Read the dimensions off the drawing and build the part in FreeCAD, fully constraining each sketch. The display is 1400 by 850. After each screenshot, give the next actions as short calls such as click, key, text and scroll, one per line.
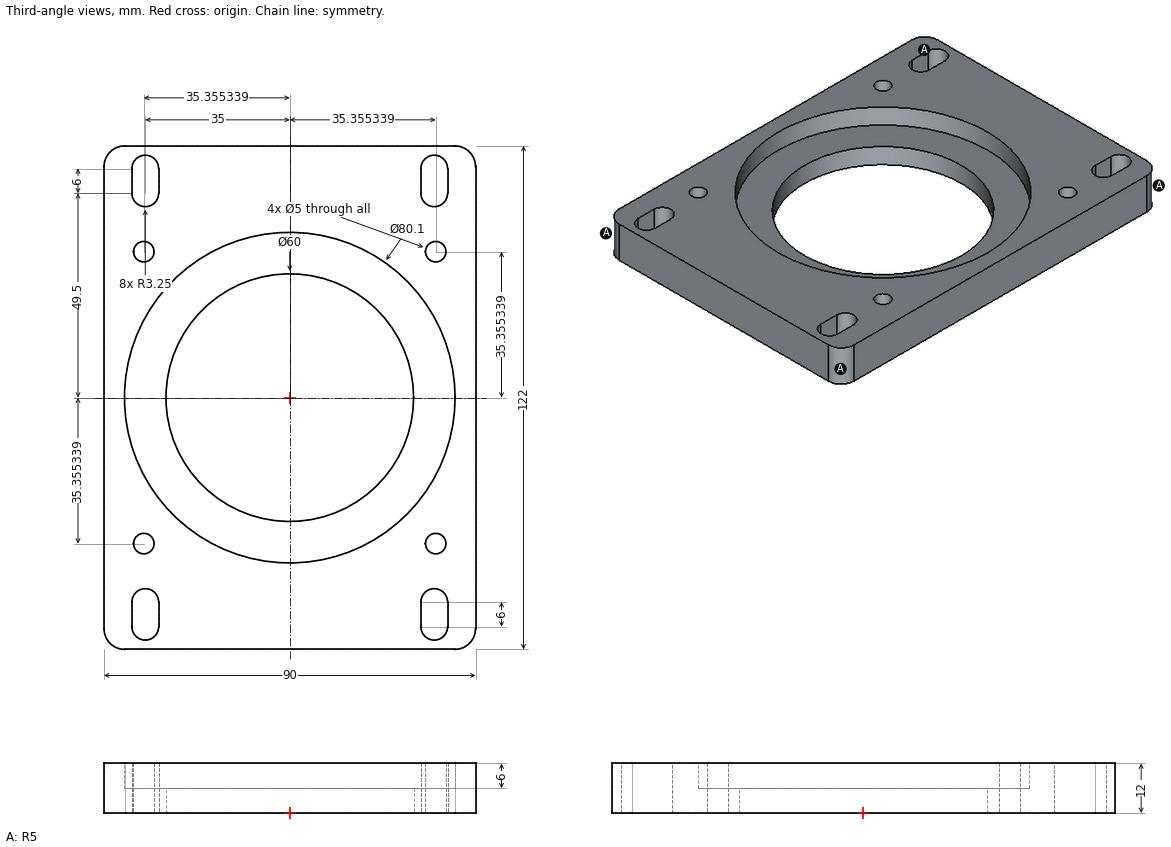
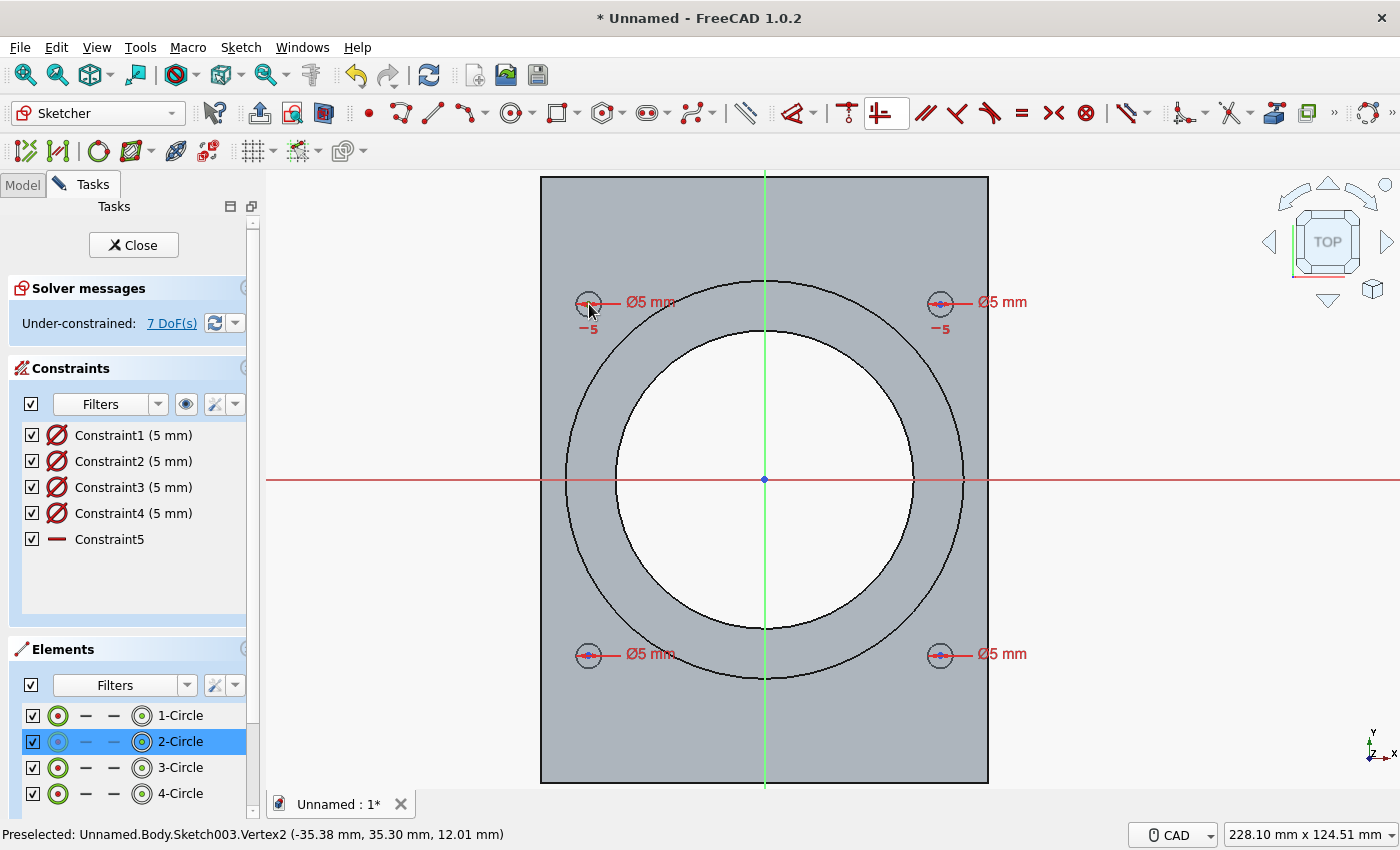
click(589, 656)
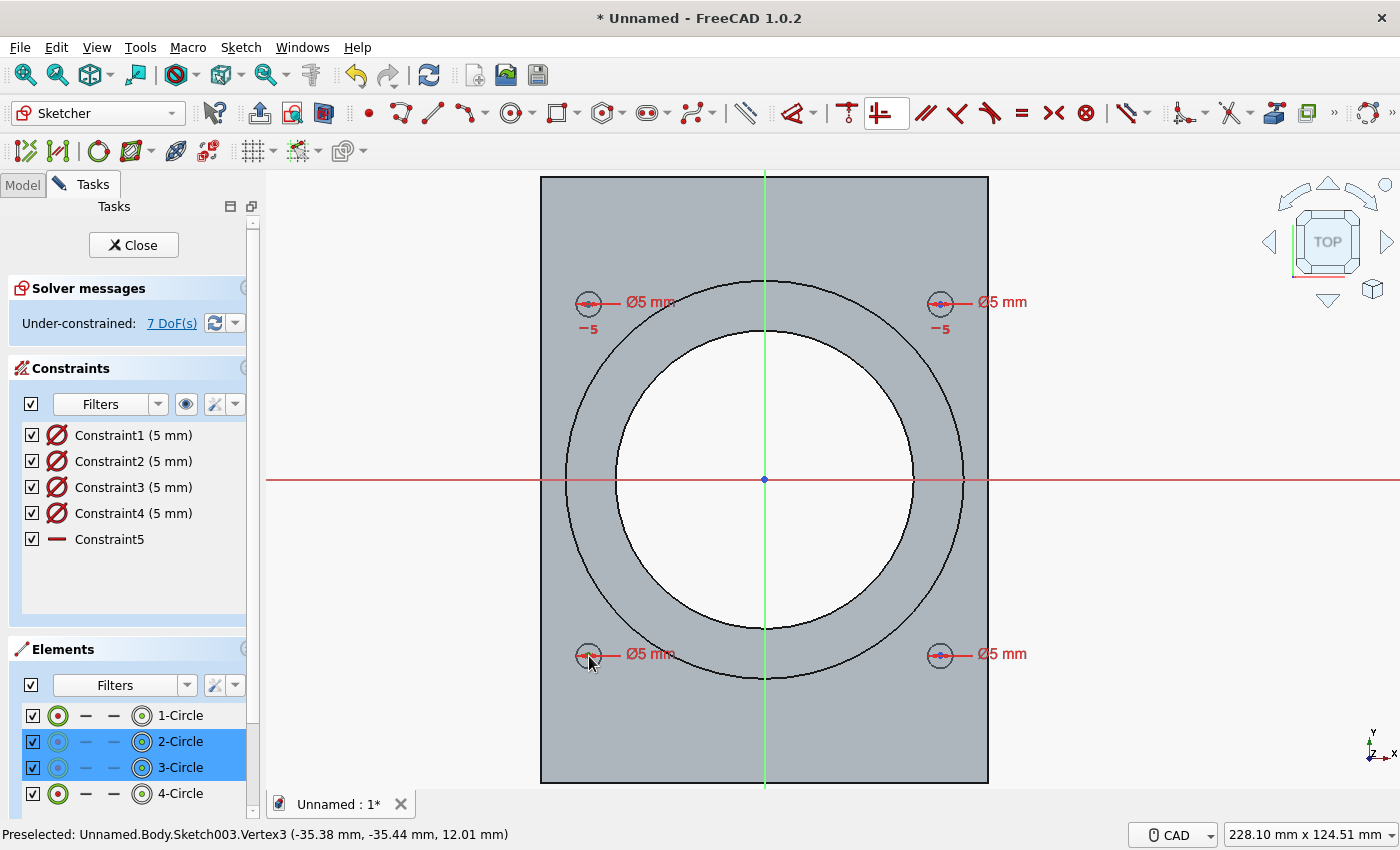
click(904, 114)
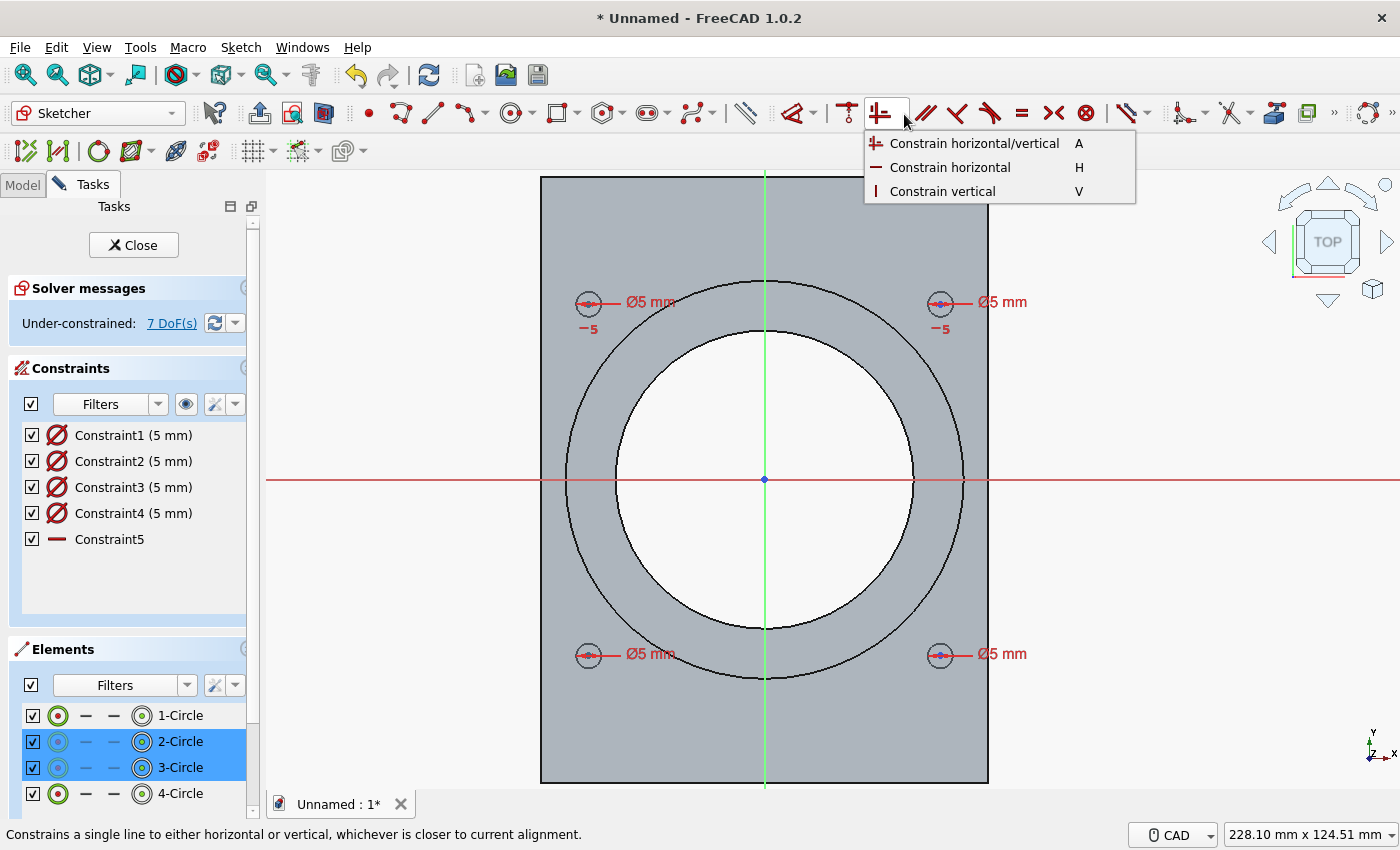
click(1000, 191)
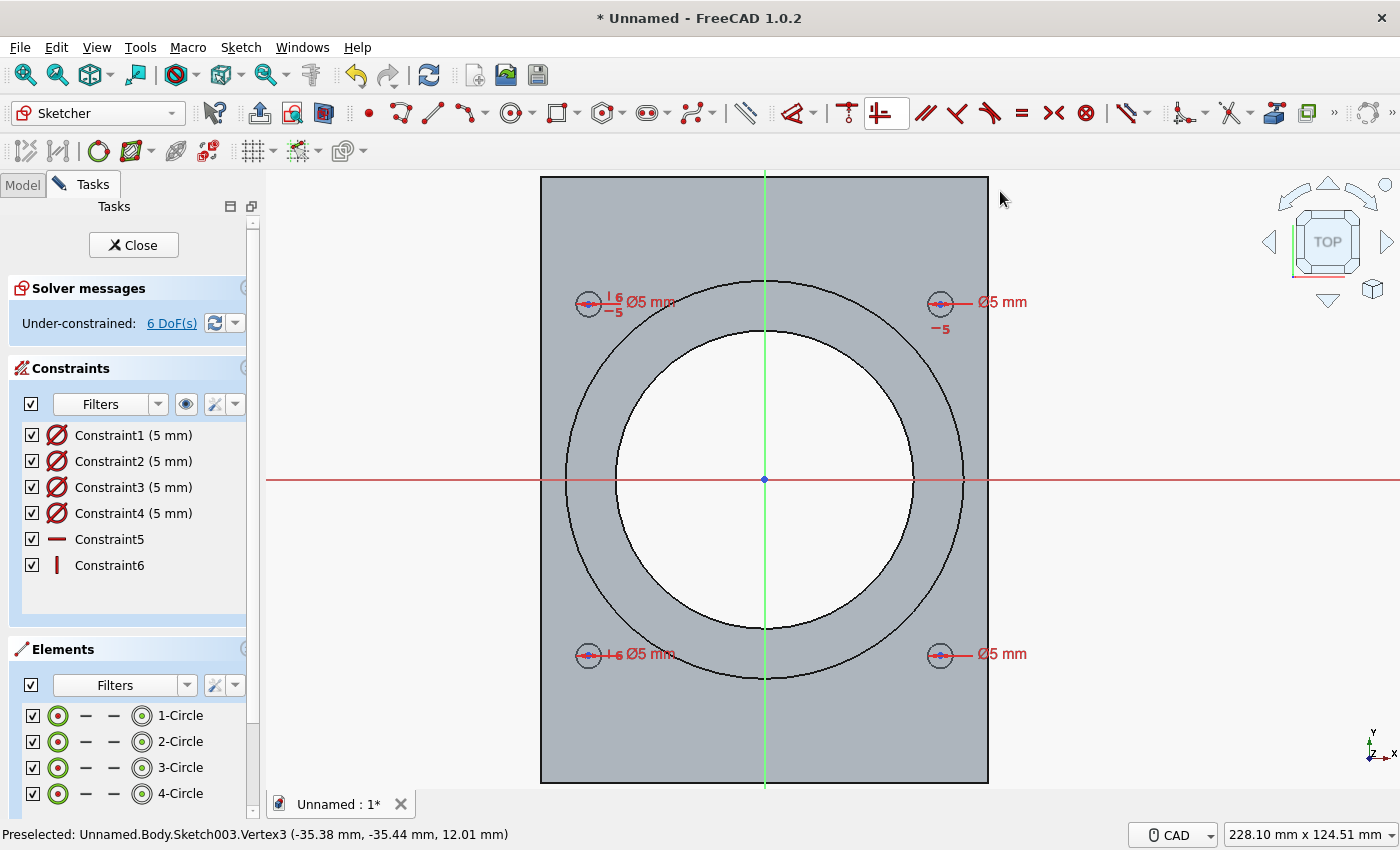
click(941, 304)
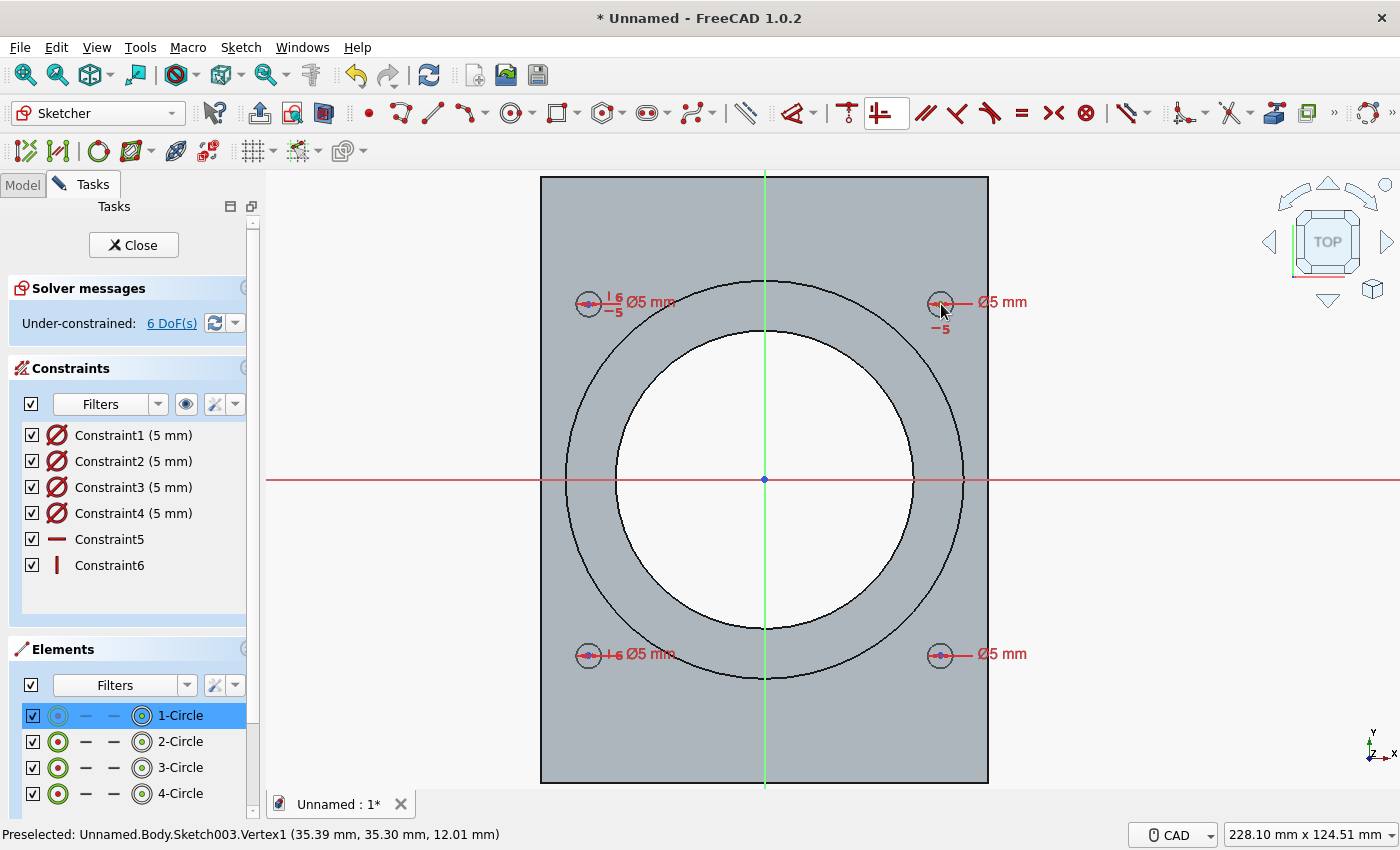
click(940, 656)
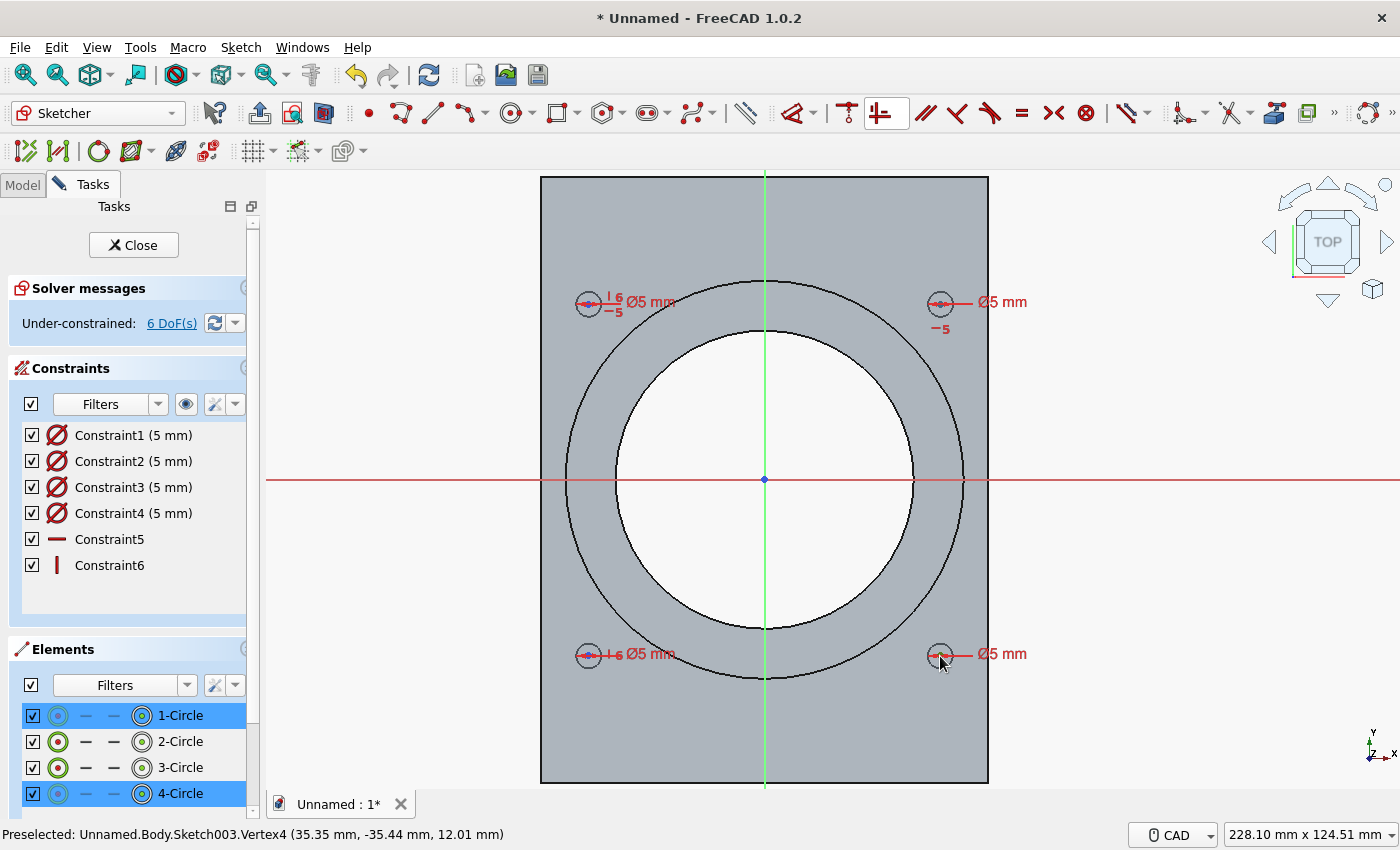
key(v)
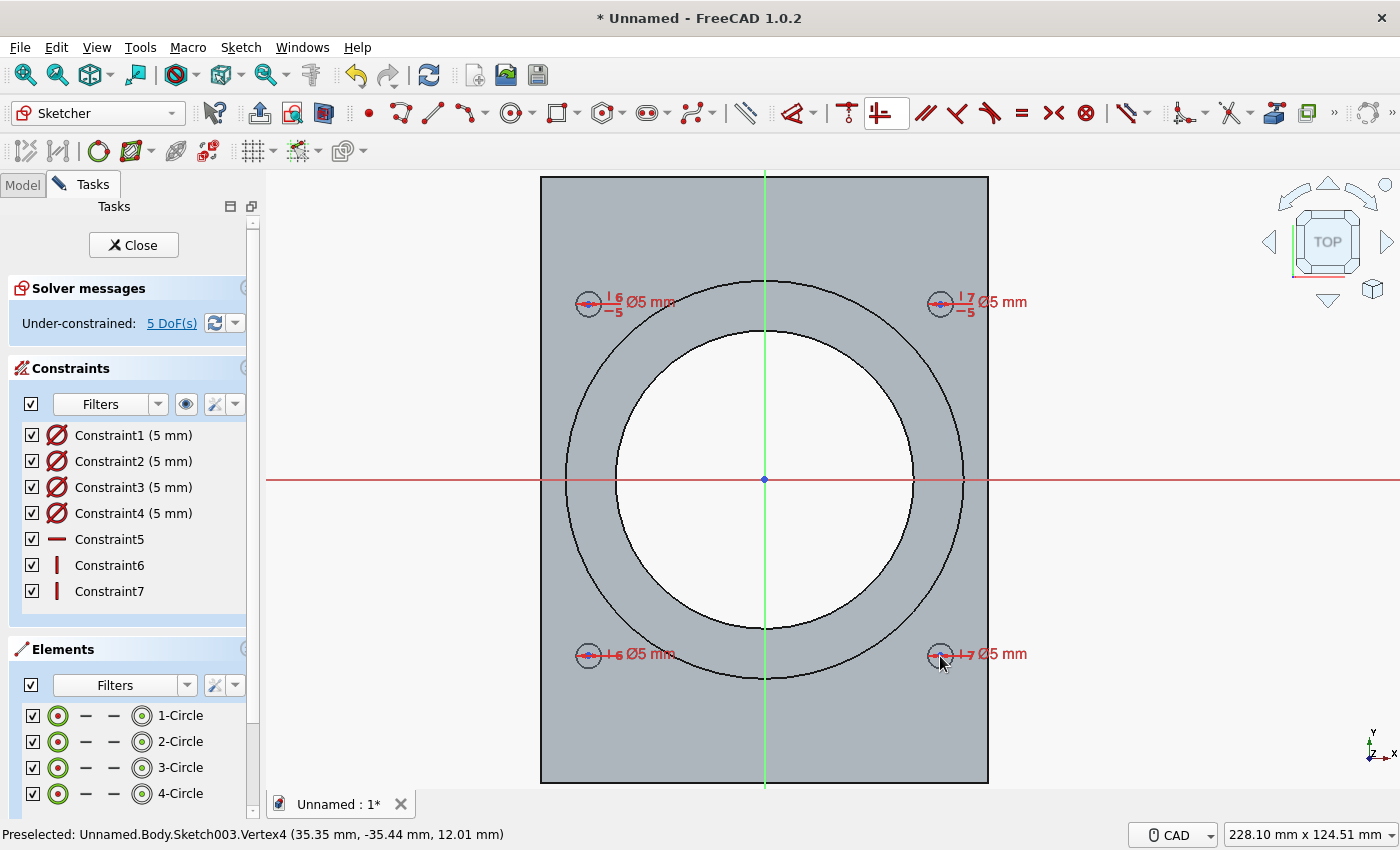
click(589, 656)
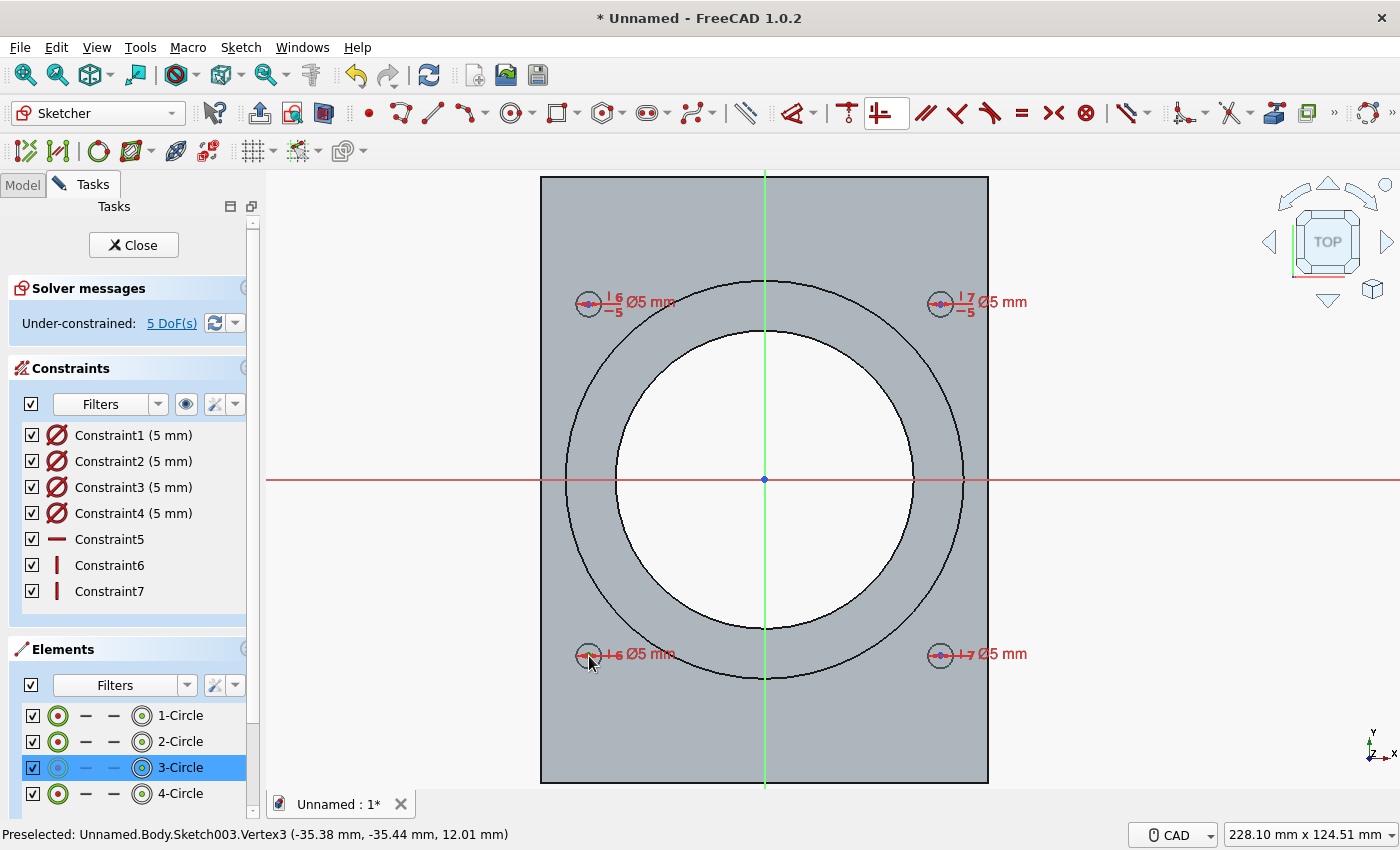
click(941, 656)